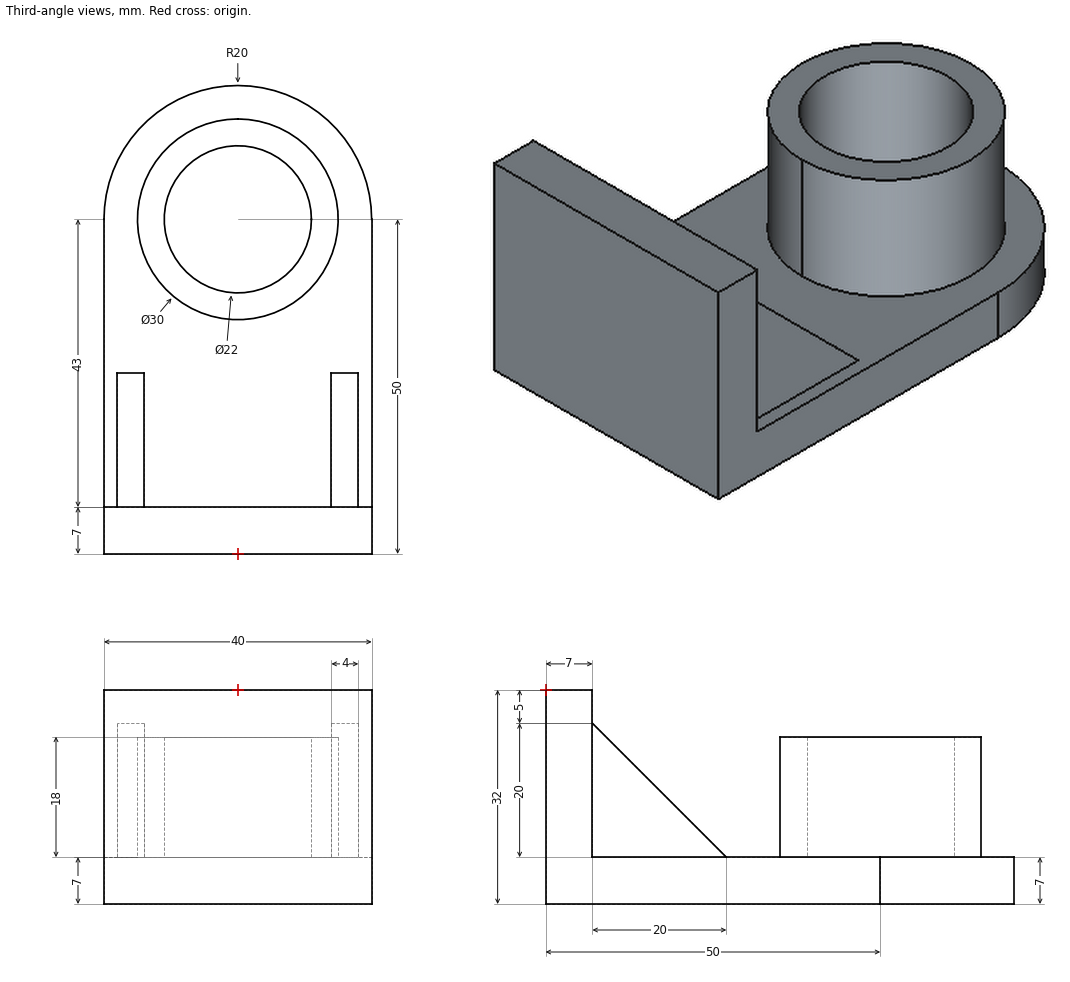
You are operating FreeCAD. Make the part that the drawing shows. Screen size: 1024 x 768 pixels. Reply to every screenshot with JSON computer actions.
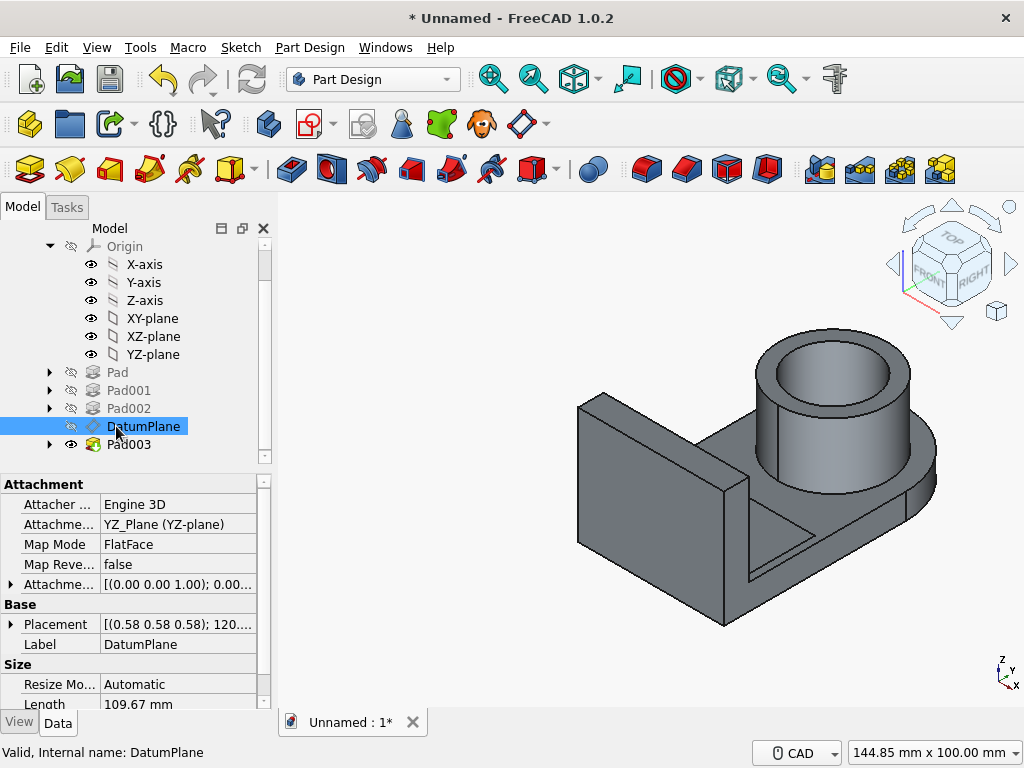
{"action": "left_click", "coordinate": [116, 444]}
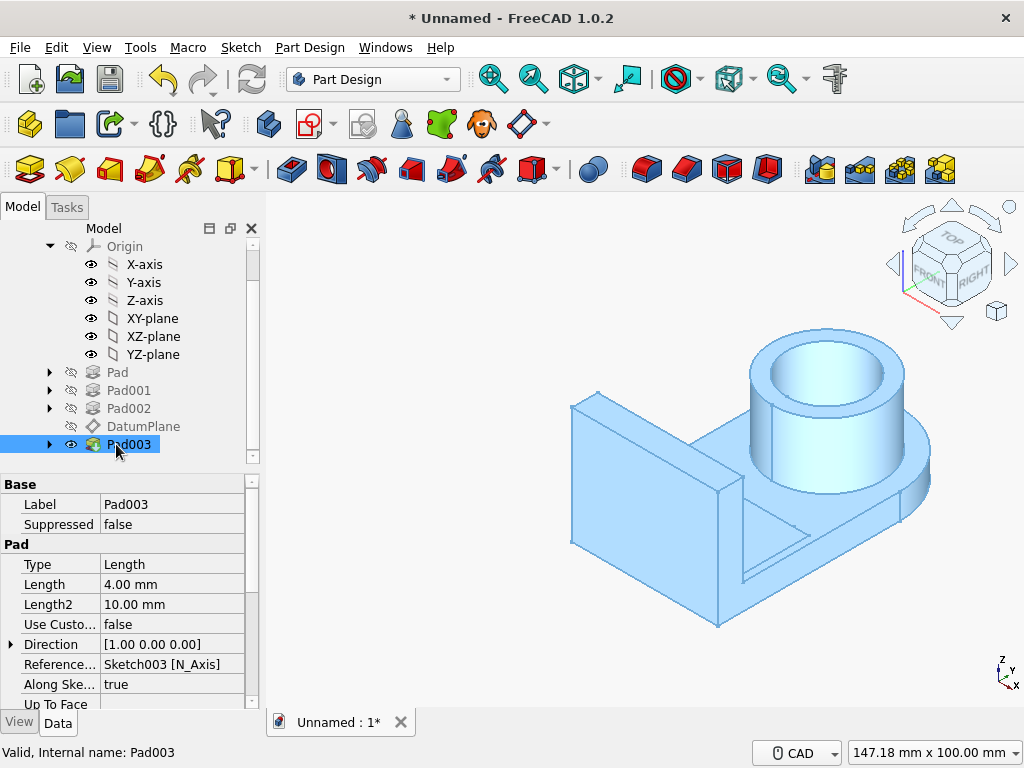
{"action": "left_click", "coordinate": [820, 170]}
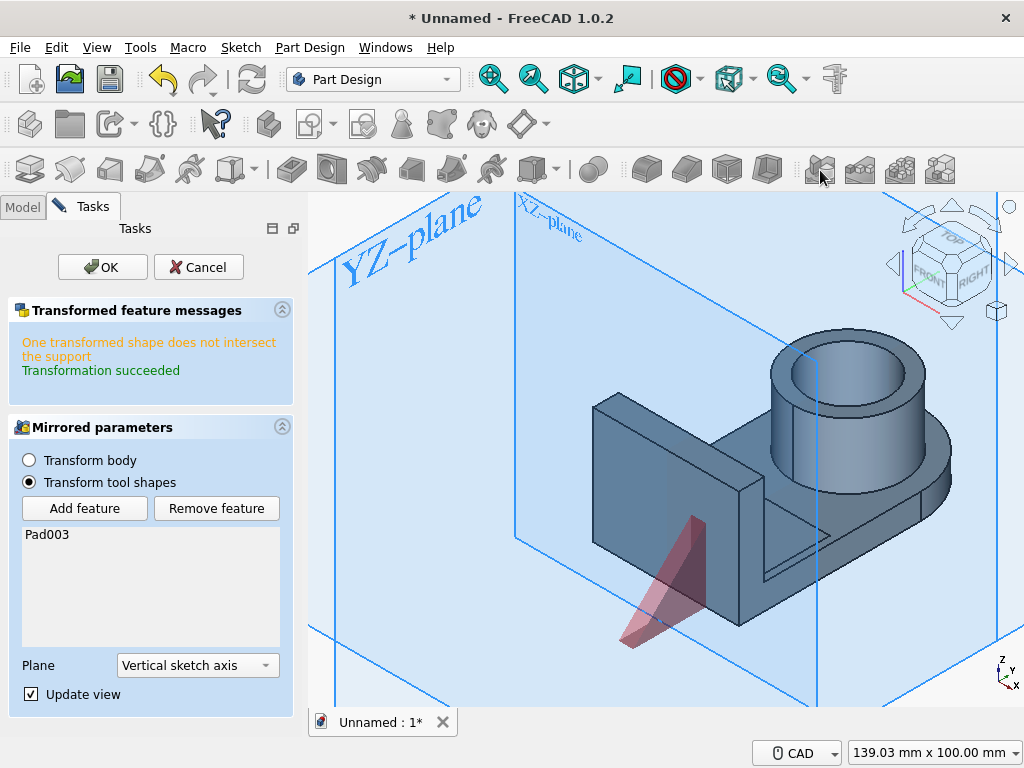
{"action": "left_click", "coordinate": [198, 666]}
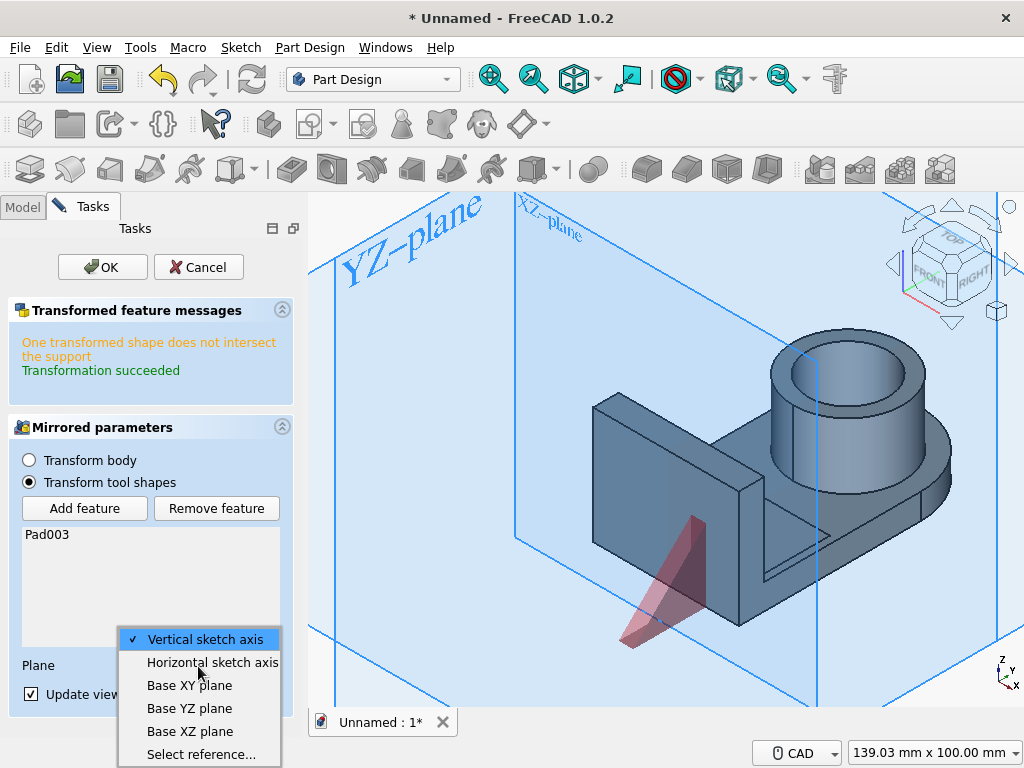
{"action": "left_click", "coordinate": [198, 708]}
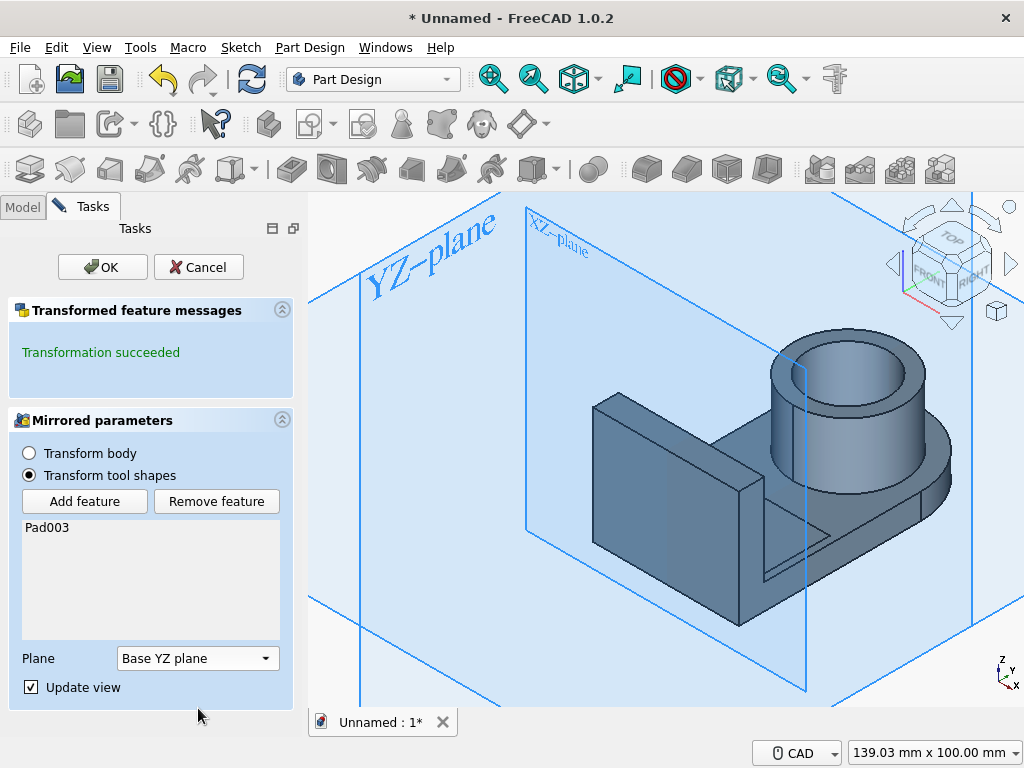
{"action": "left_click", "coordinate": [103, 267]}